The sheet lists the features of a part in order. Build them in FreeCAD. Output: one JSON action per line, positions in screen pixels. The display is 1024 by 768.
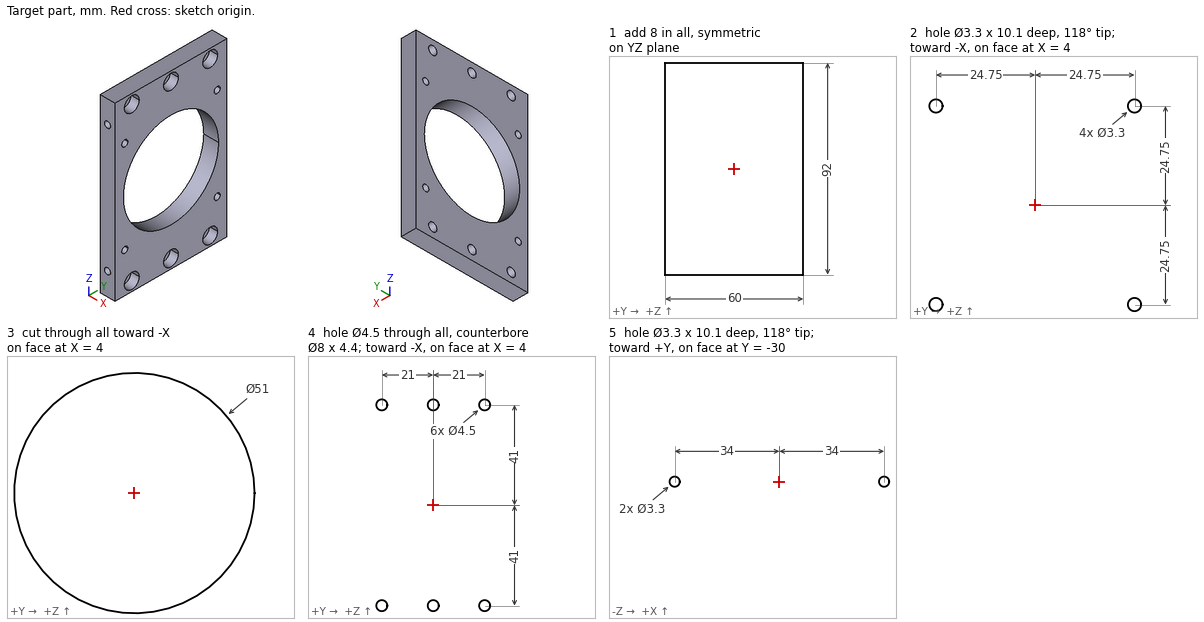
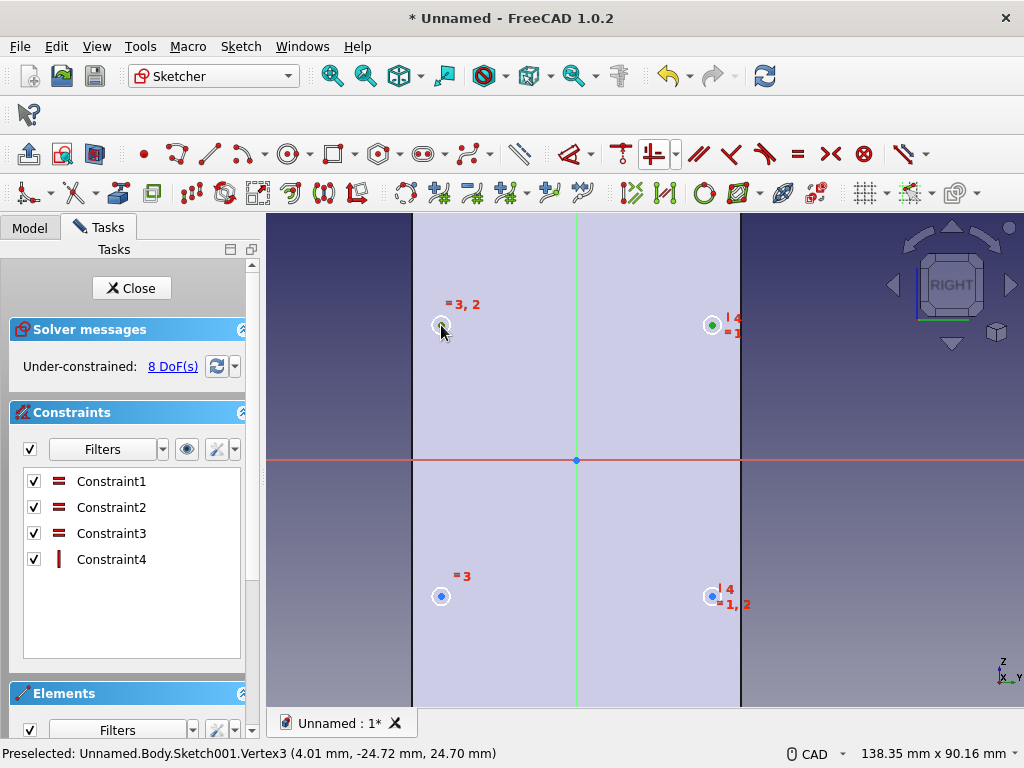
{"action": "left_click", "coordinate": [676, 154]}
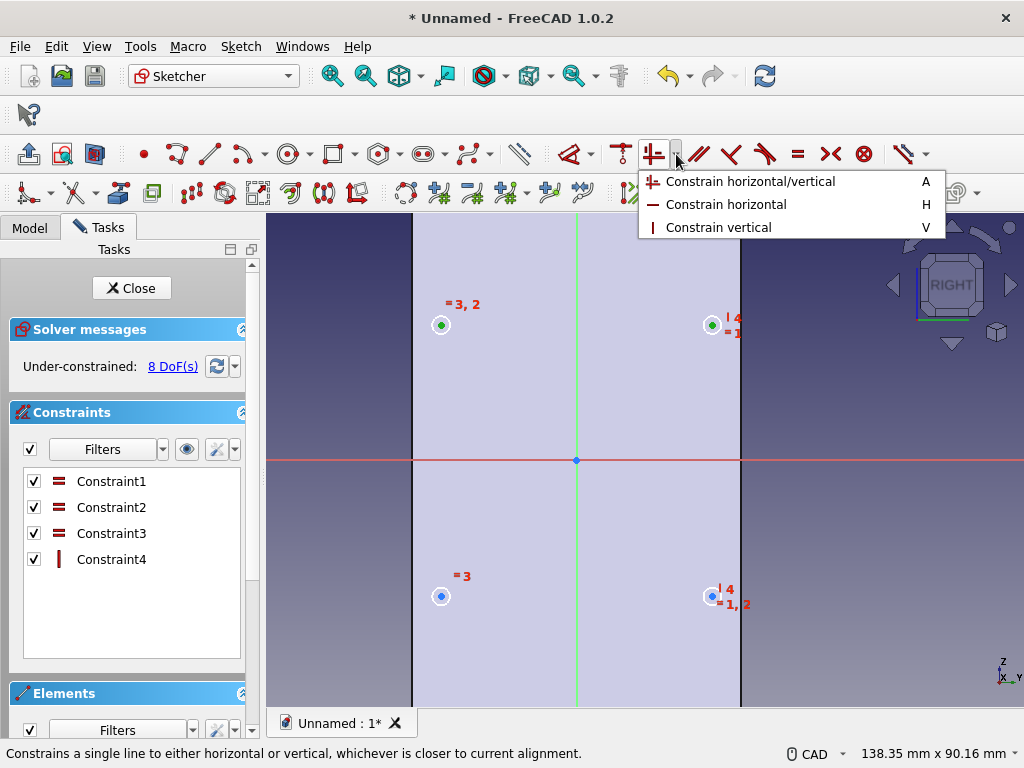
{"action": "left_click", "coordinate": [792, 204]}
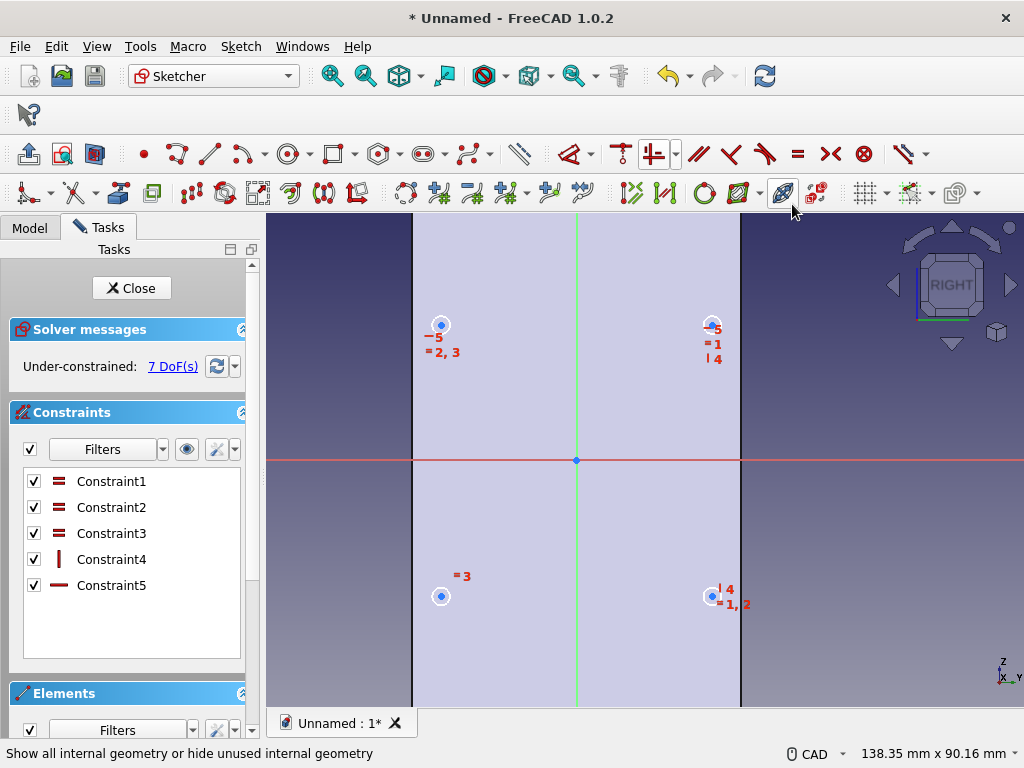
{"action": "left_click", "coordinate": [441, 325]}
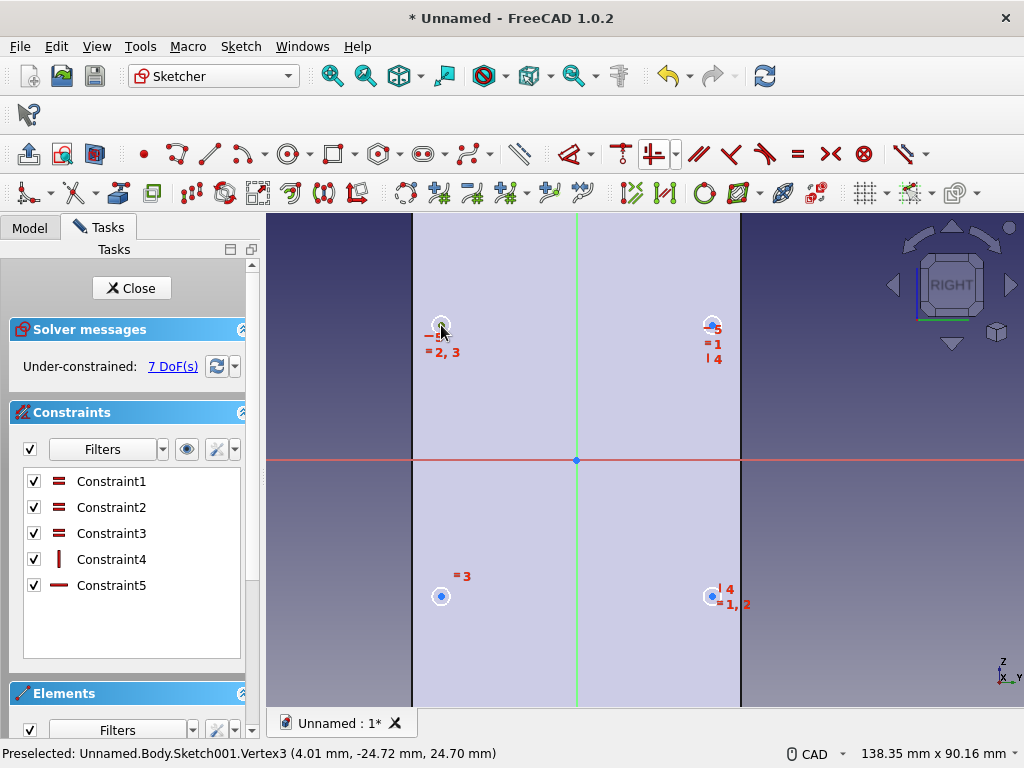
{"action": "left_click", "coordinate": [441, 596]}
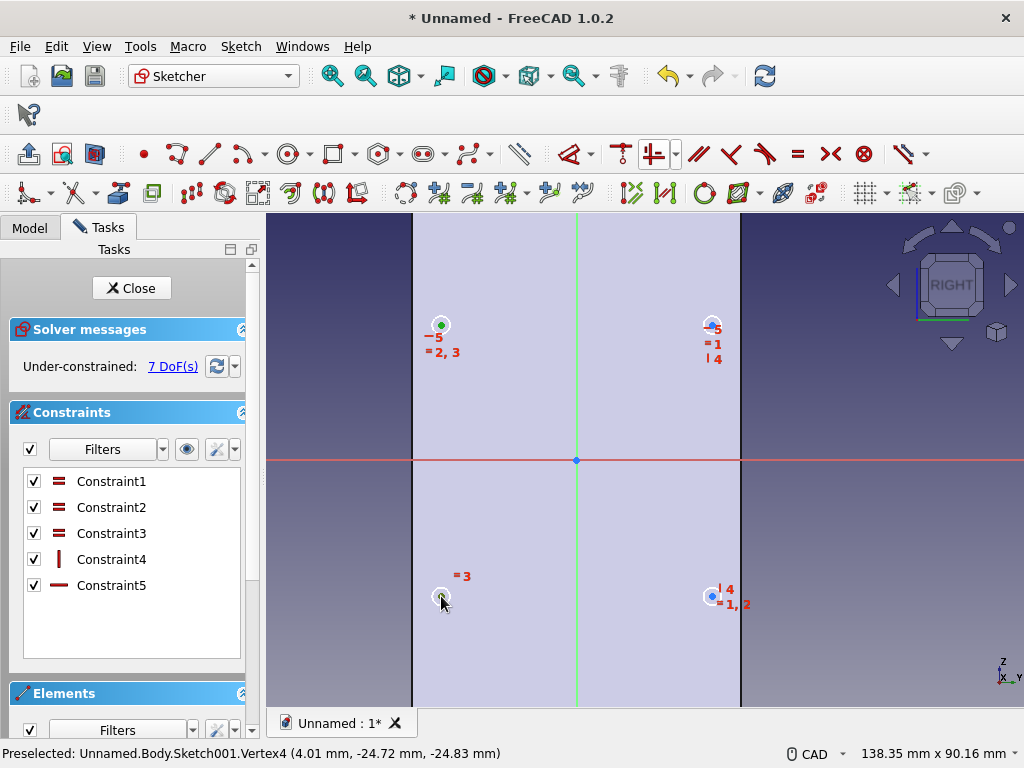
{"action": "left_click", "coordinate": [676, 154]}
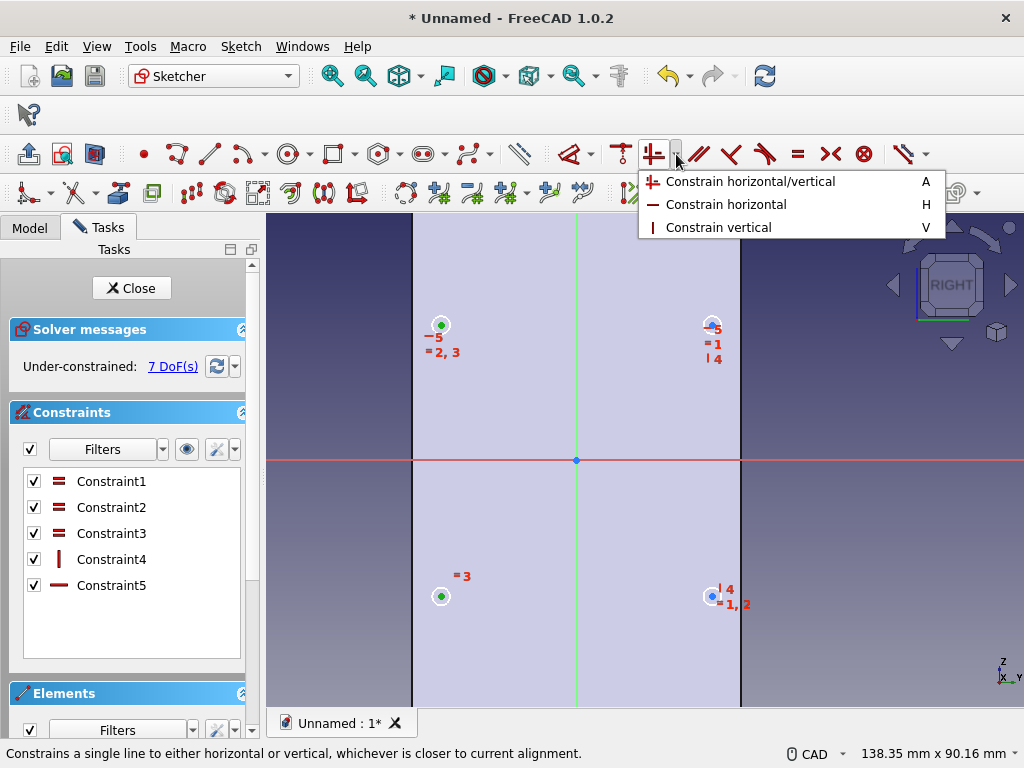
{"action": "left_click", "coordinate": [792, 228]}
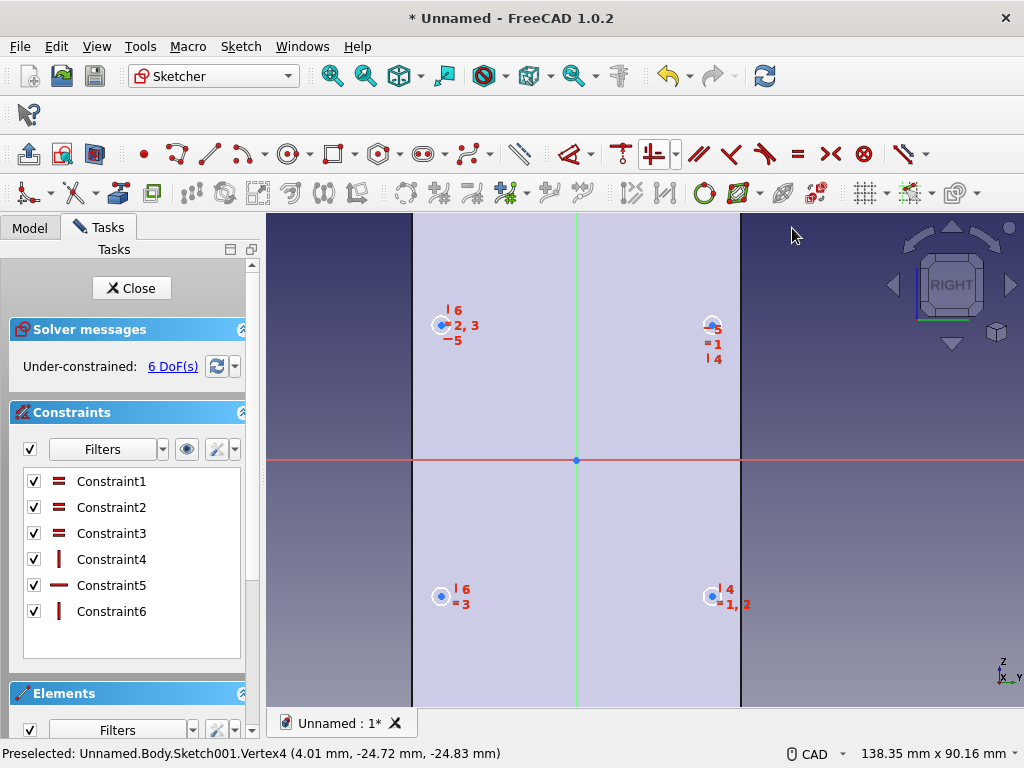
{"action": "left_click", "coordinate": [712, 596]}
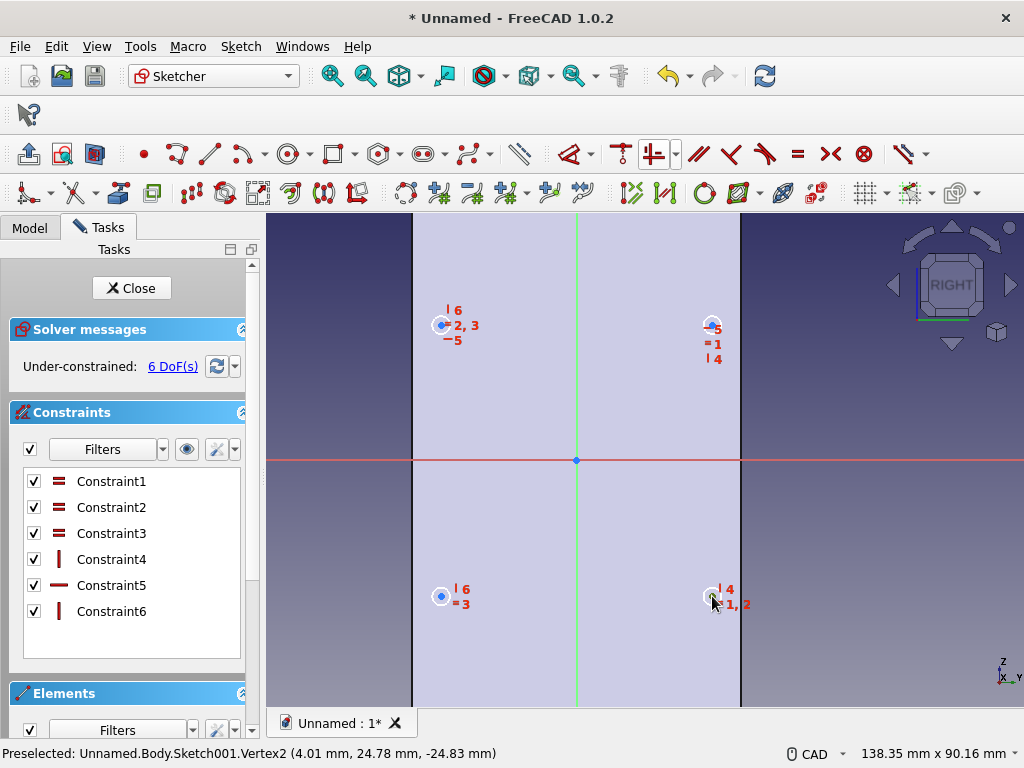
{"action": "left_click", "coordinate": [441, 596]}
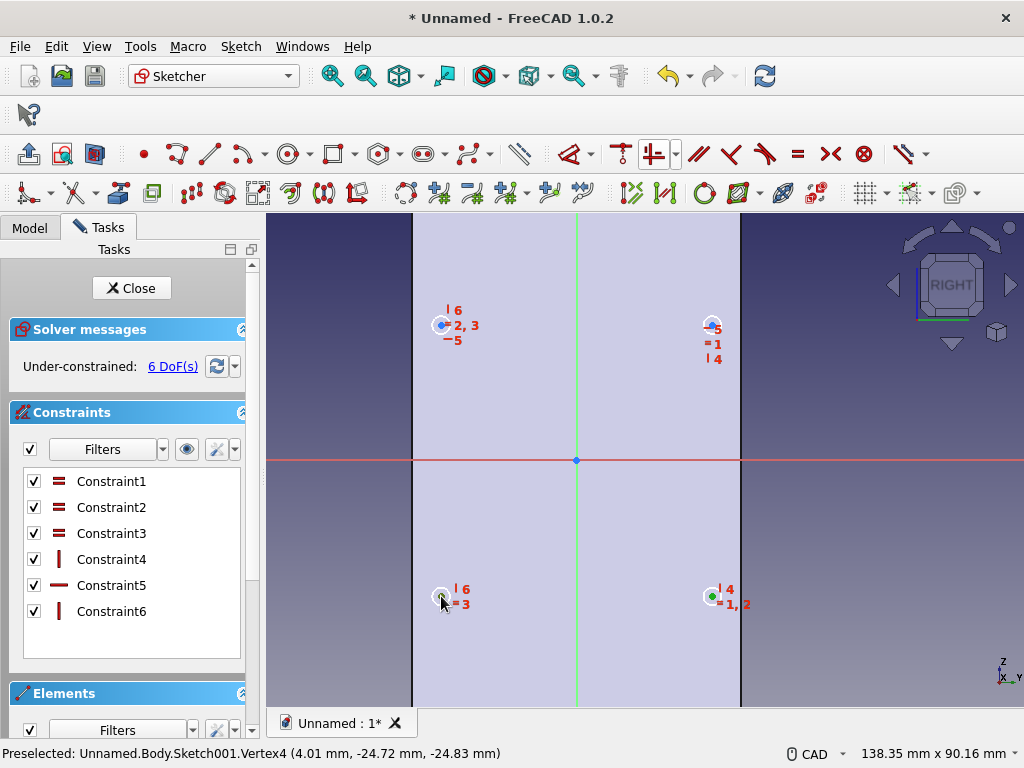
{"action": "left_click", "coordinate": [676, 154]}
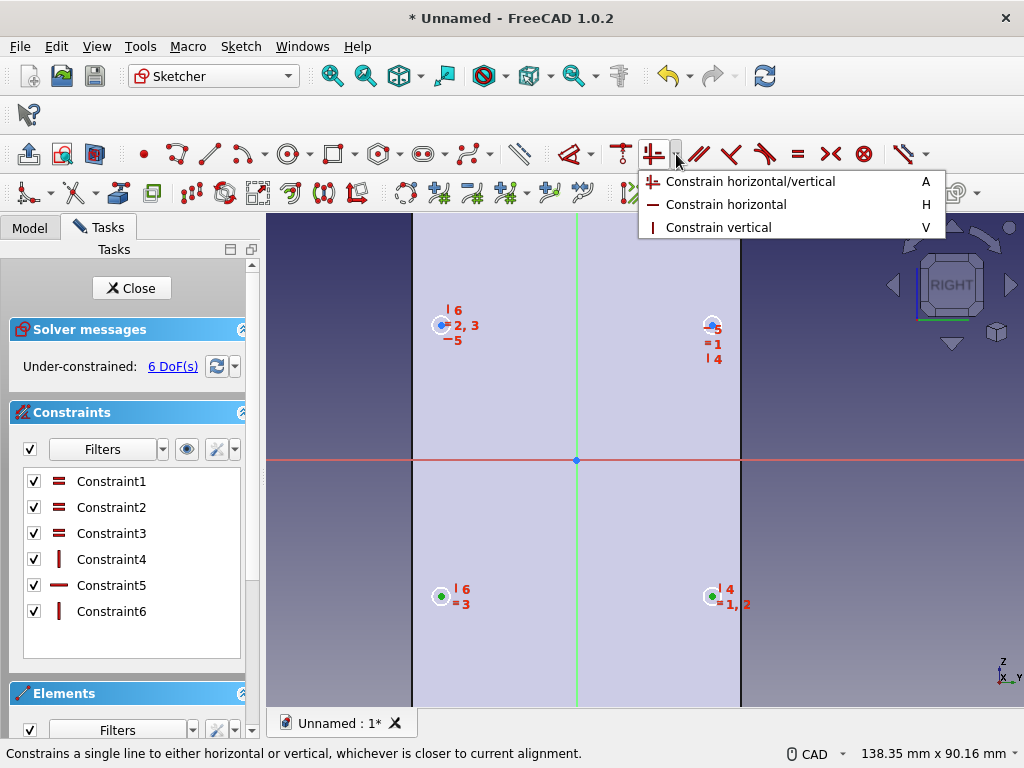
{"action": "left_click", "coordinate": [792, 204]}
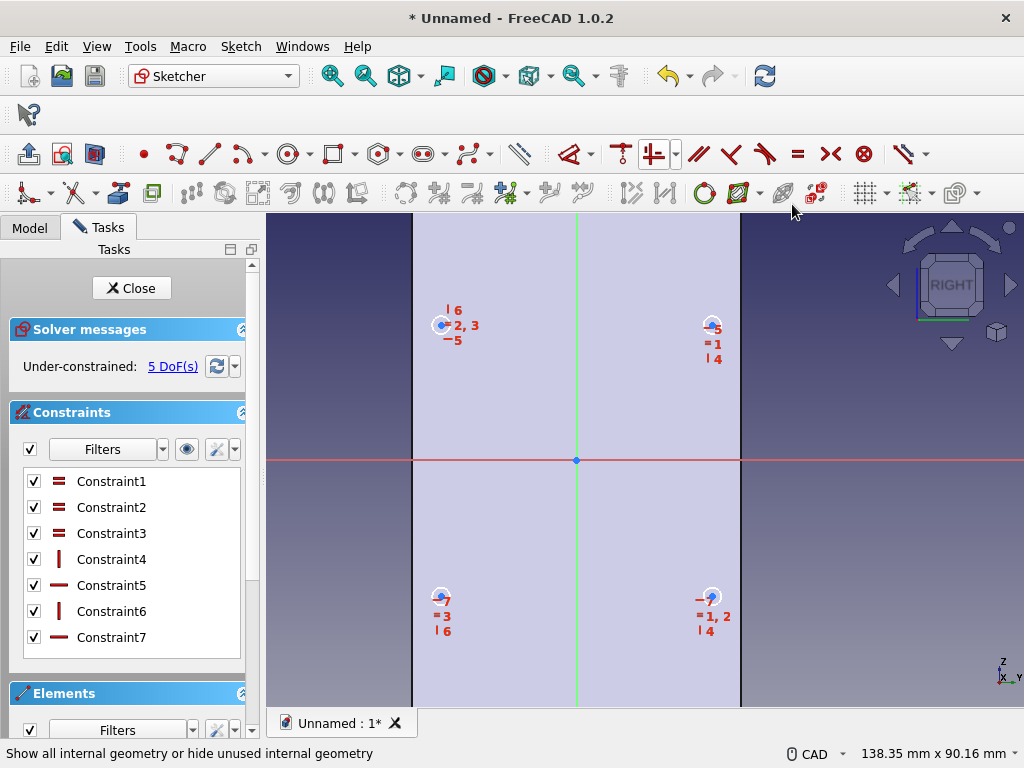
{"action": "left_click", "coordinate": [568, 154]}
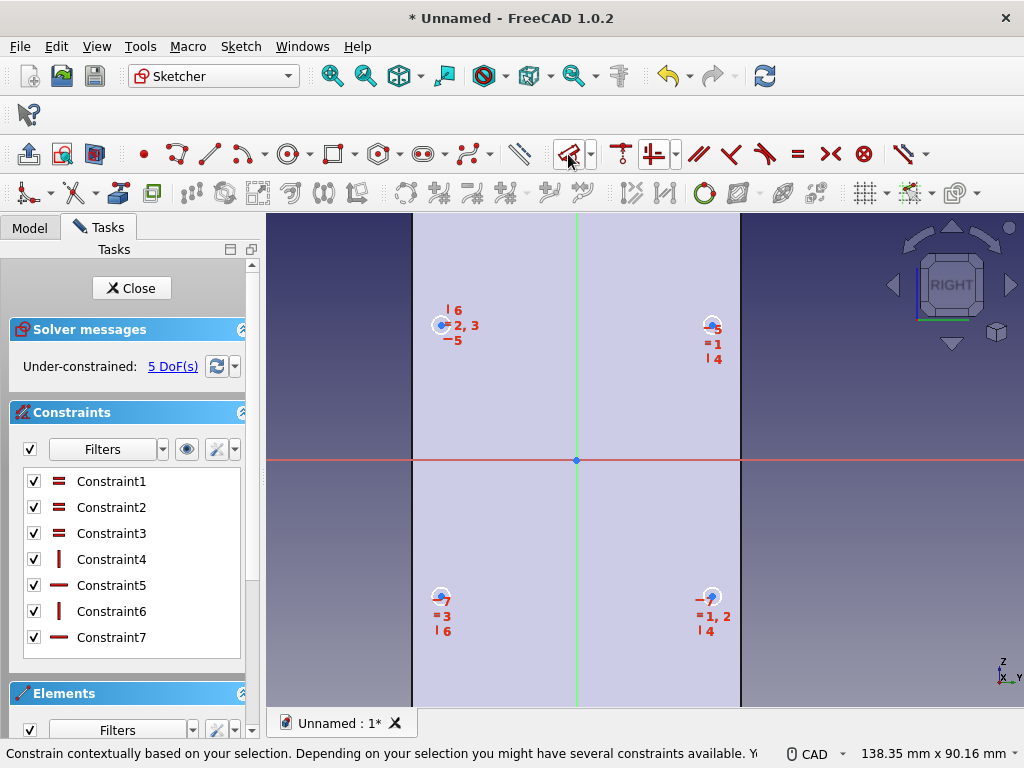
{"action": "scroll", "coordinate": [713, 316], "scroll_direction": "up", "scroll_amount": 4}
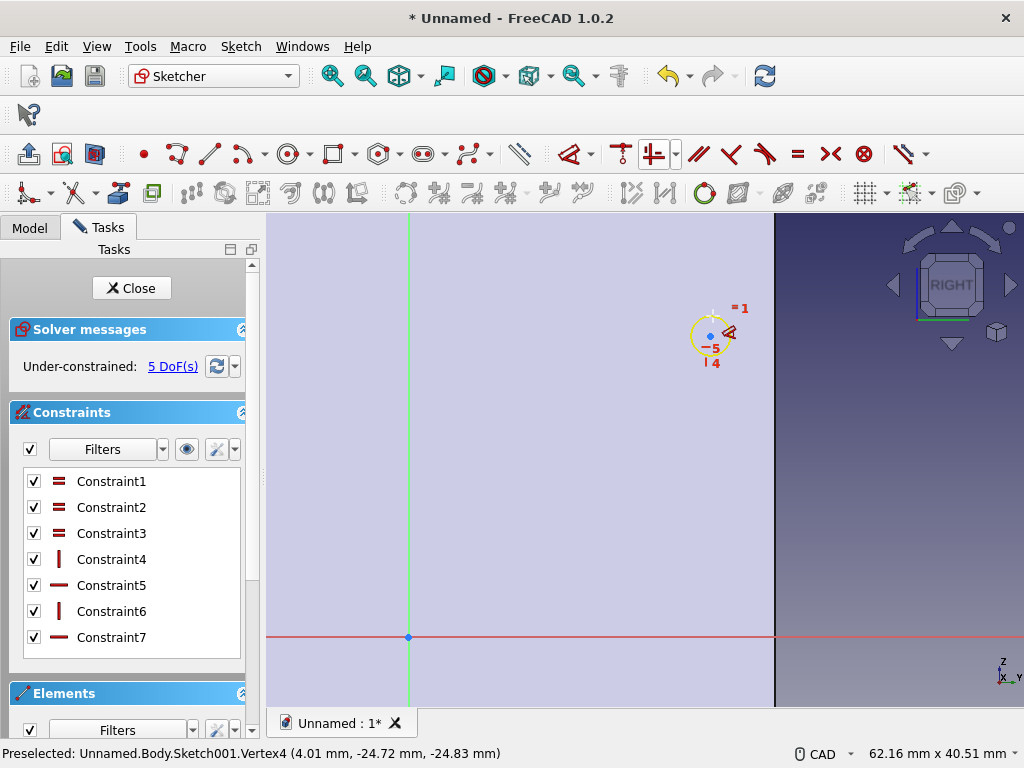
{"action": "left_click", "coordinate": [711, 316]}
{"action": "left_click", "coordinate": [711, 284]}